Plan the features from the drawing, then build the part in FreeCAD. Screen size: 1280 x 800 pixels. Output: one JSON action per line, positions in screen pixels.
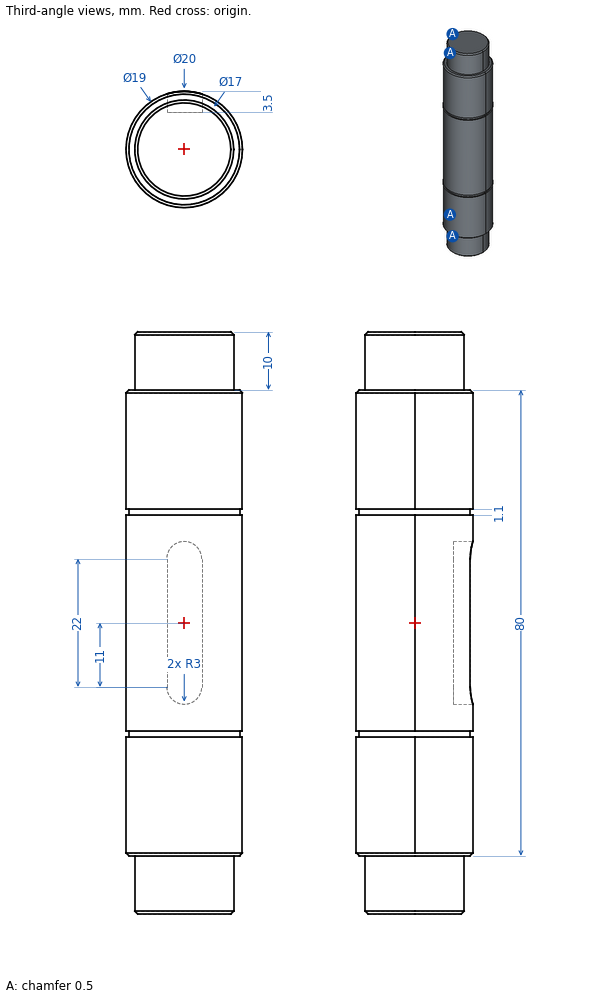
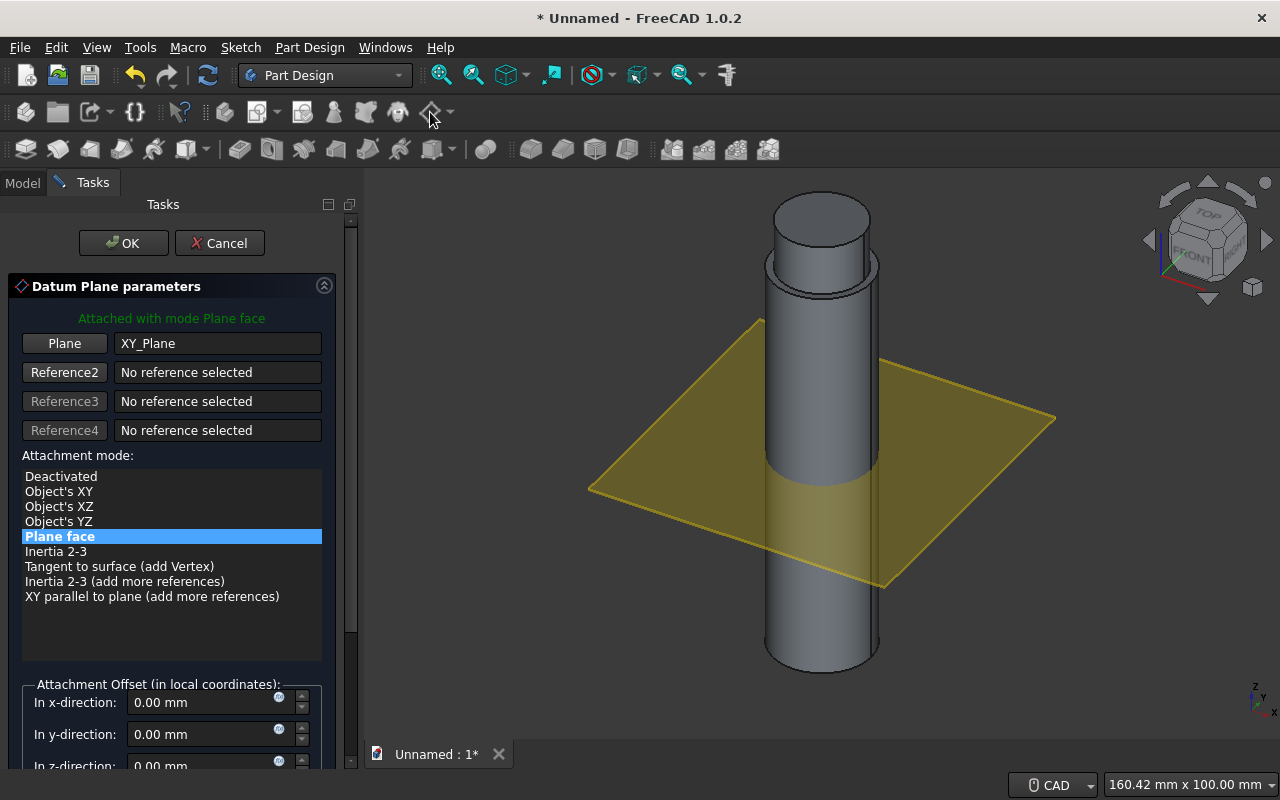
{"action": "scroll", "coordinate": [351, 491], "scroll_direction": "down", "scroll_amount": 2}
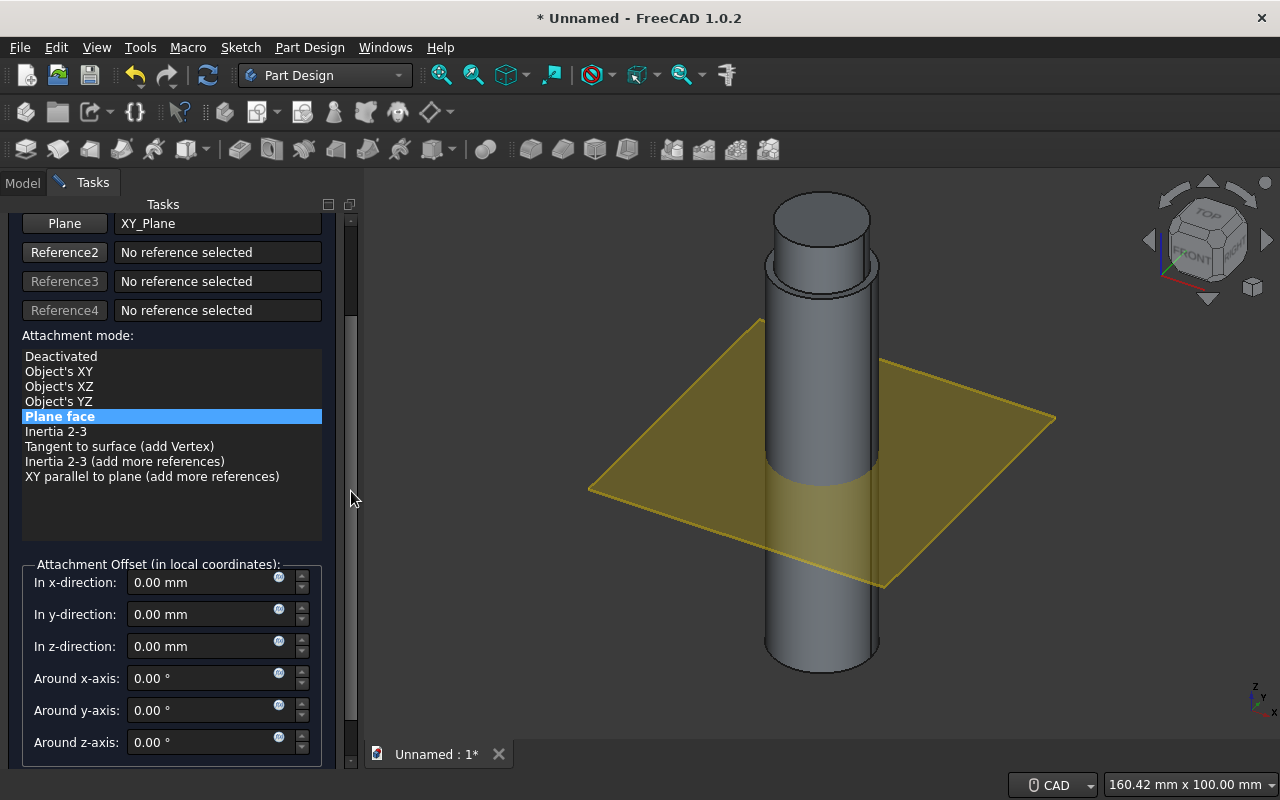
{"action": "triple_click", "coordinate": [210, 646]}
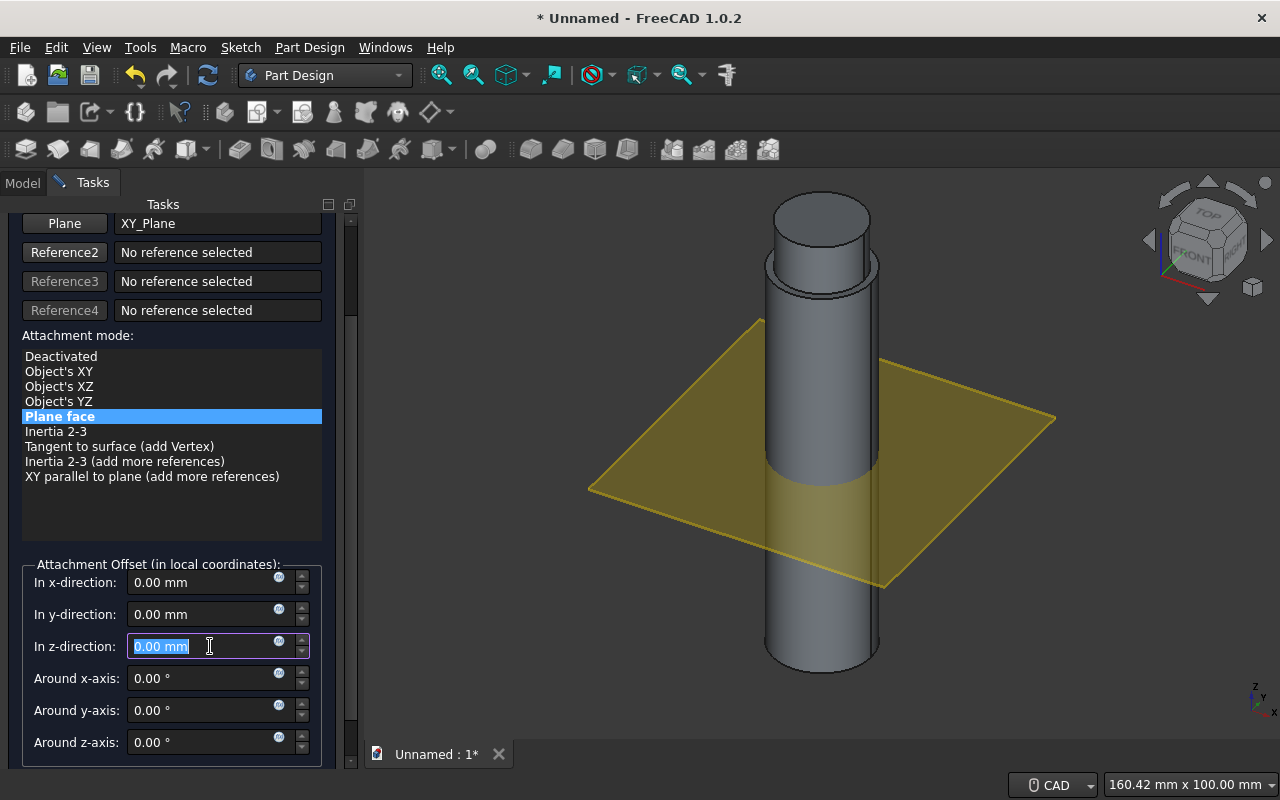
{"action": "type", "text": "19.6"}
{"action": "key", "text": "Tab"}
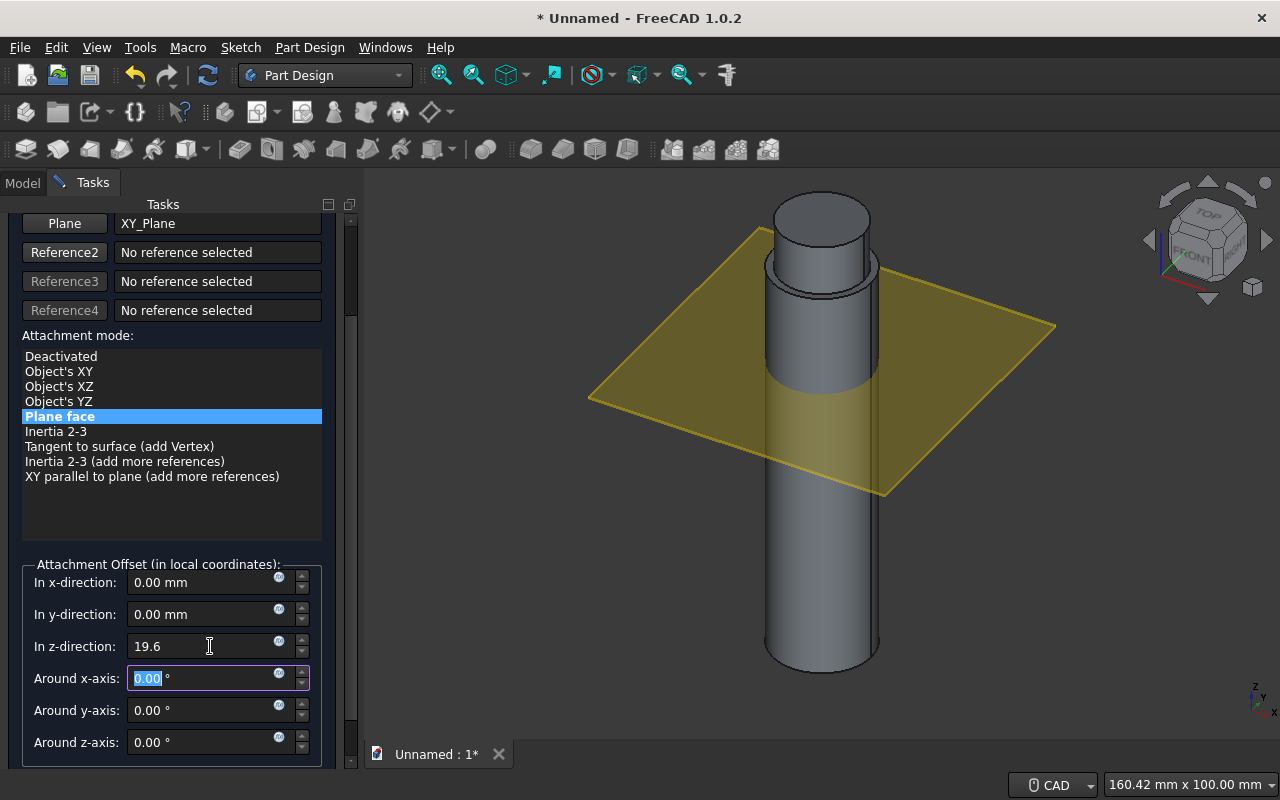
{"action": "scroll", "coordinate": [351, 491], "scroll_direction": "up", "scroll_amount": 3}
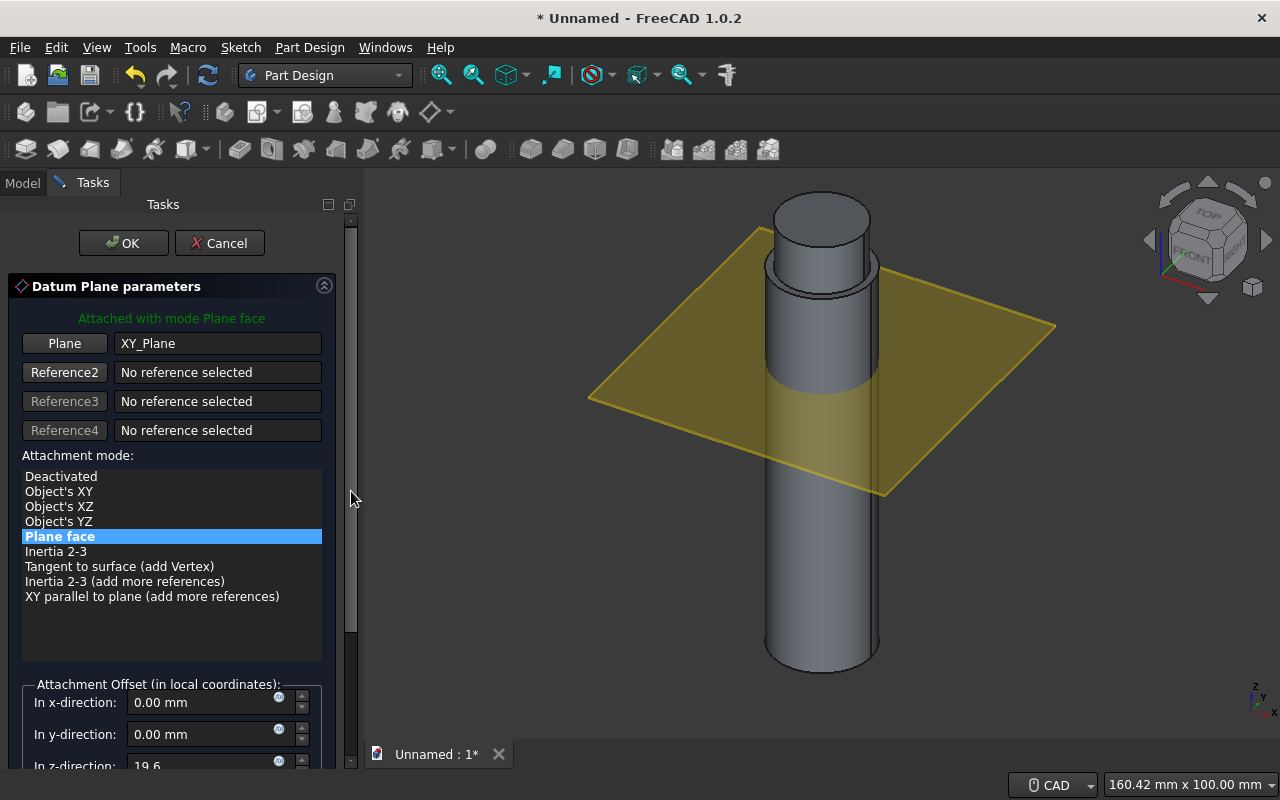
{"action": "left_click", "coordinate": [124, 243]}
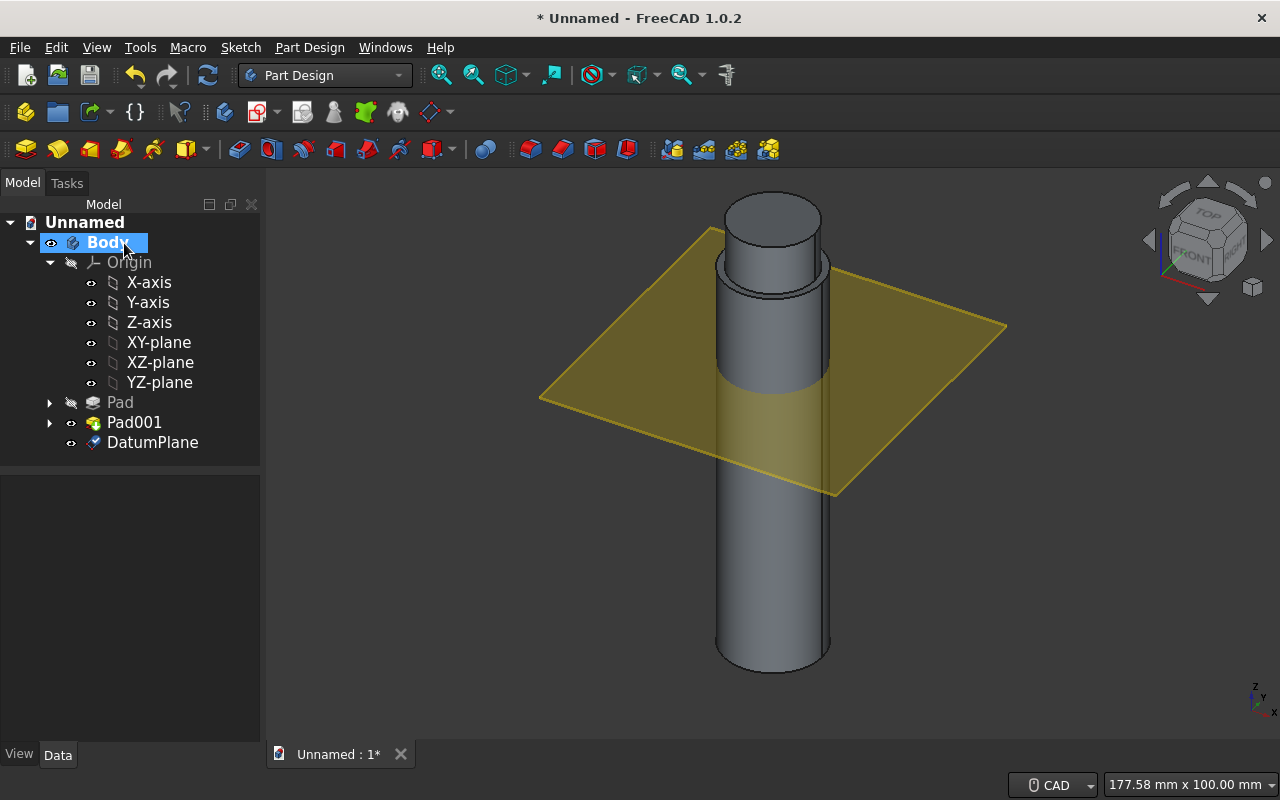
{"action": "left_click", "coordinate": [116, 443]}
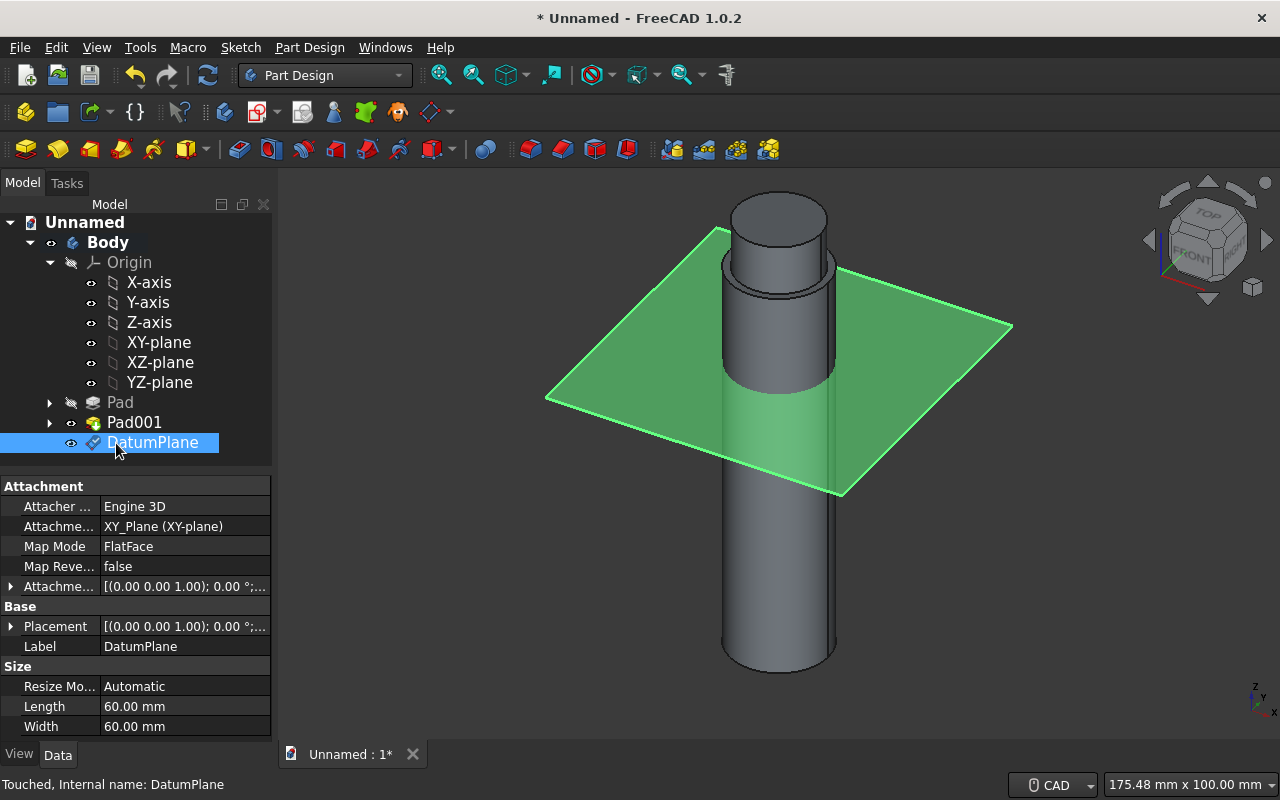
{"action": "left_click", "coordinate": [258, 112]}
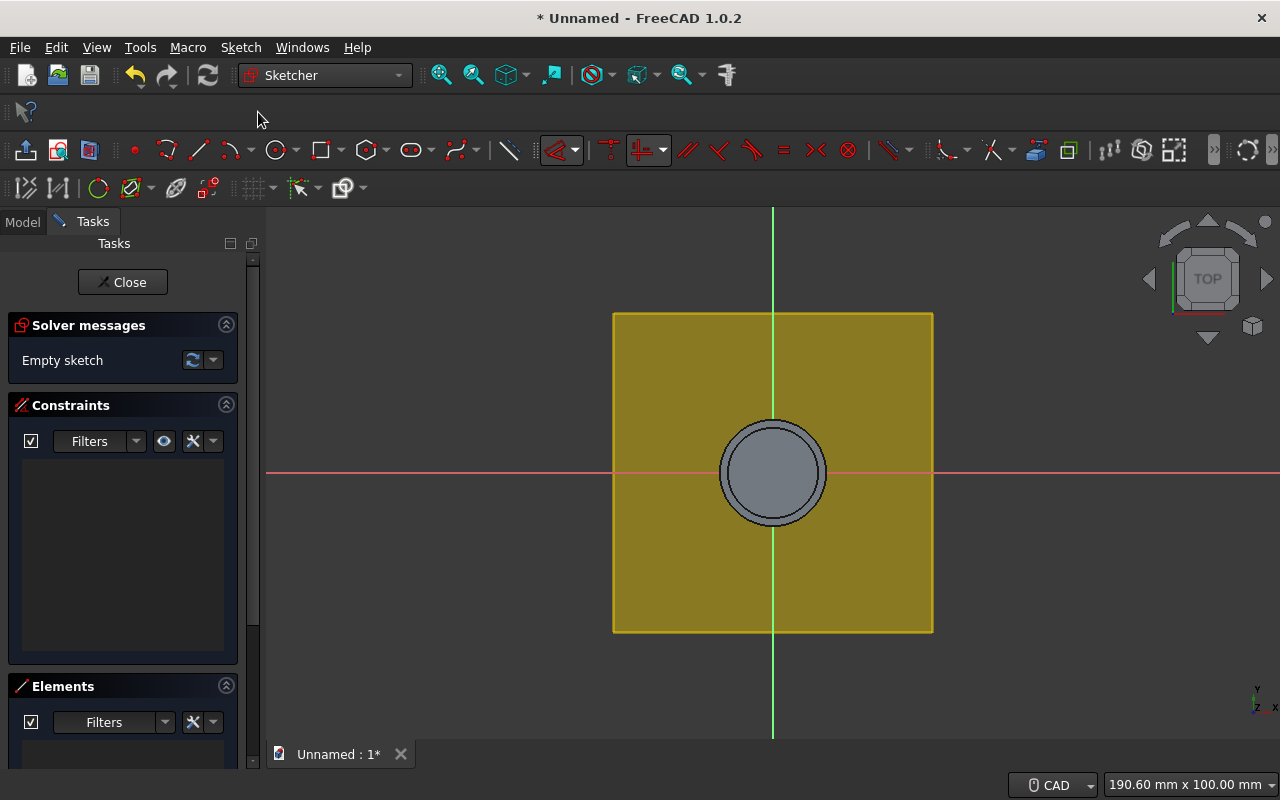
{"action": "left_click", "coordinate": [90, 150]}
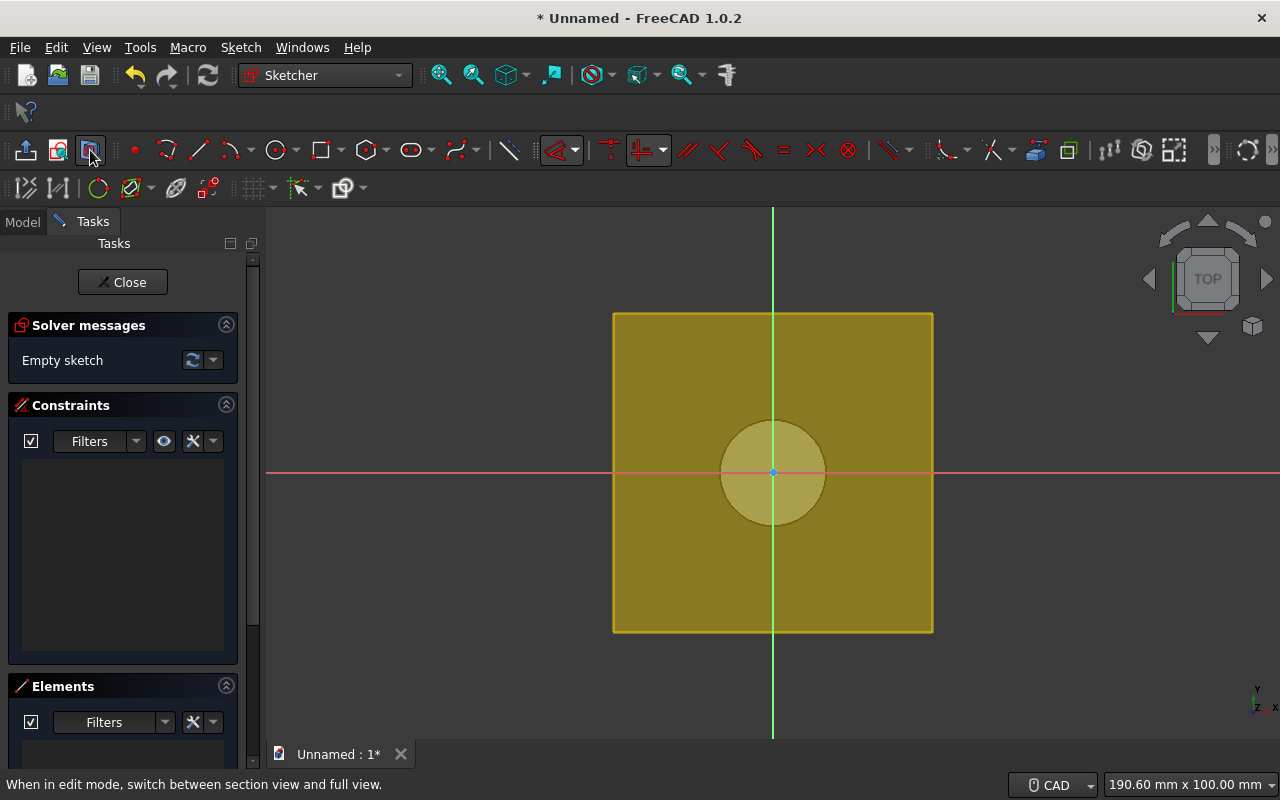
{"action": "scroll", "coordinate": [803, 473], "scroll_direction": "up", "scroll_amount": 6}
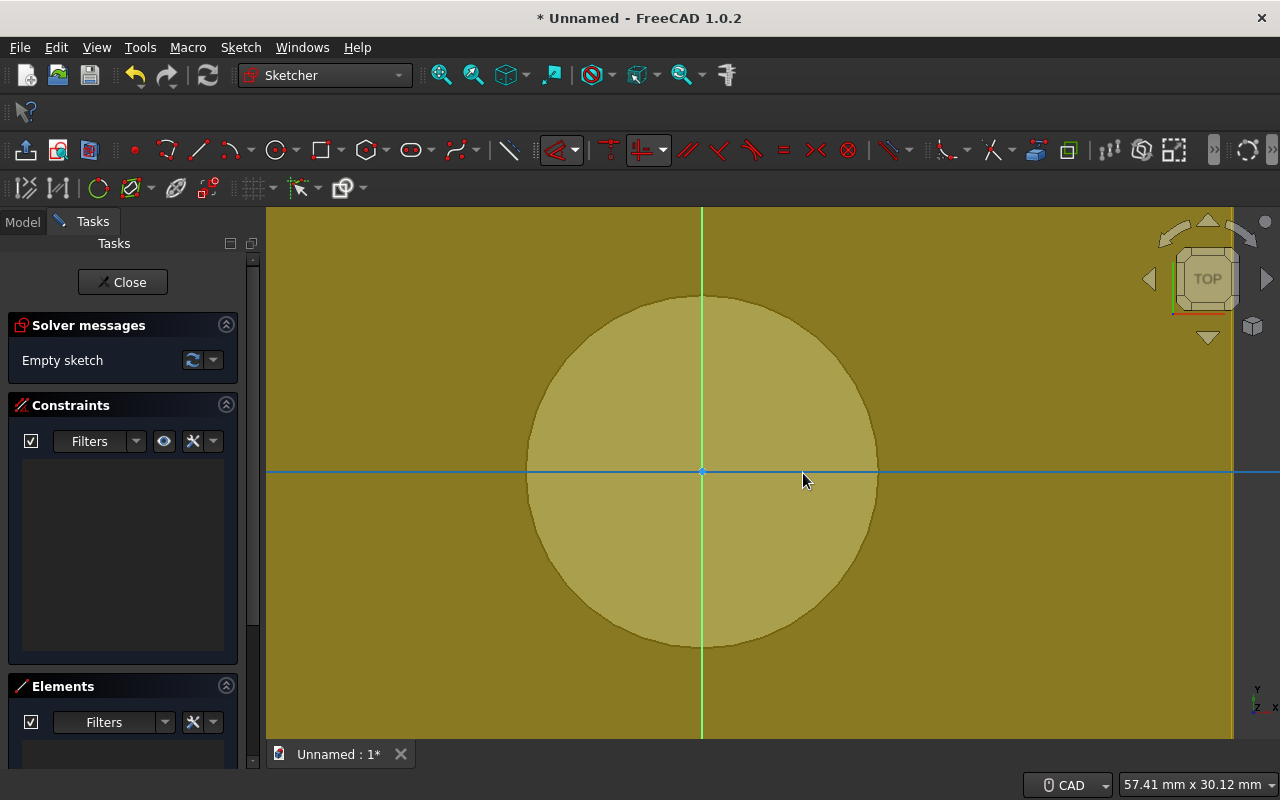
{"action": "left_click", "coordinate": [276, 150]}